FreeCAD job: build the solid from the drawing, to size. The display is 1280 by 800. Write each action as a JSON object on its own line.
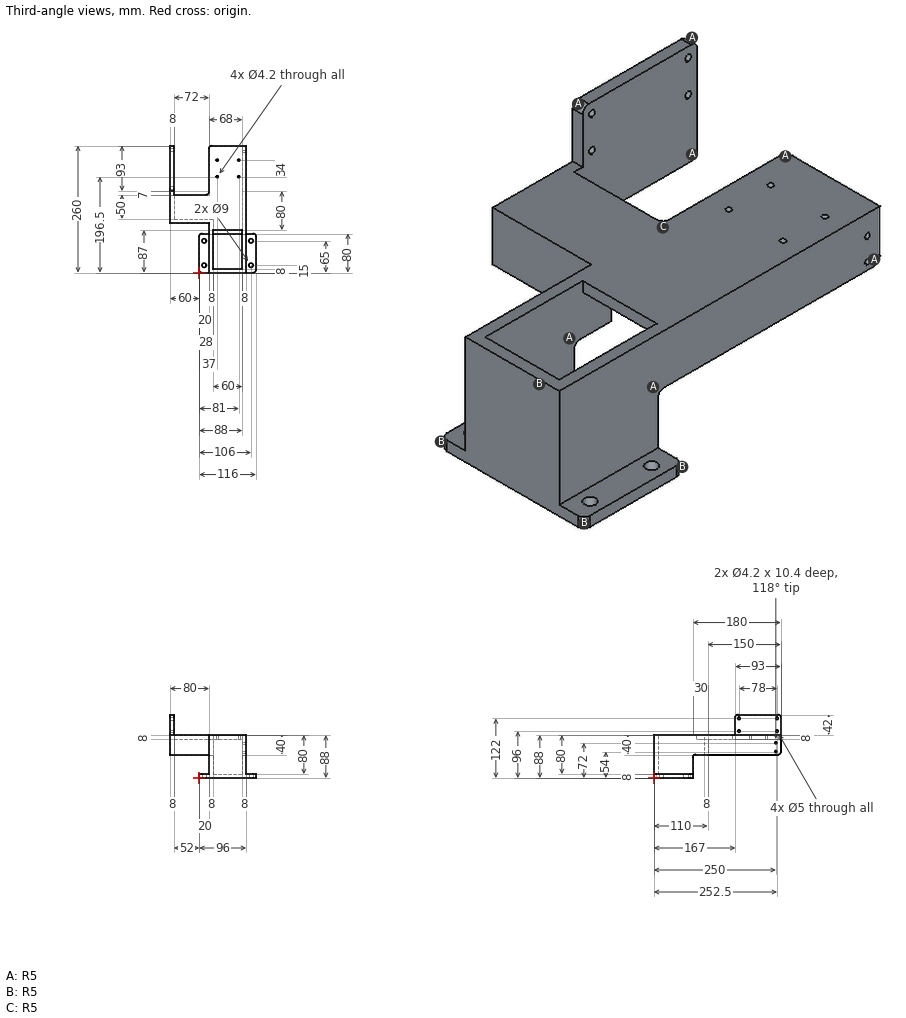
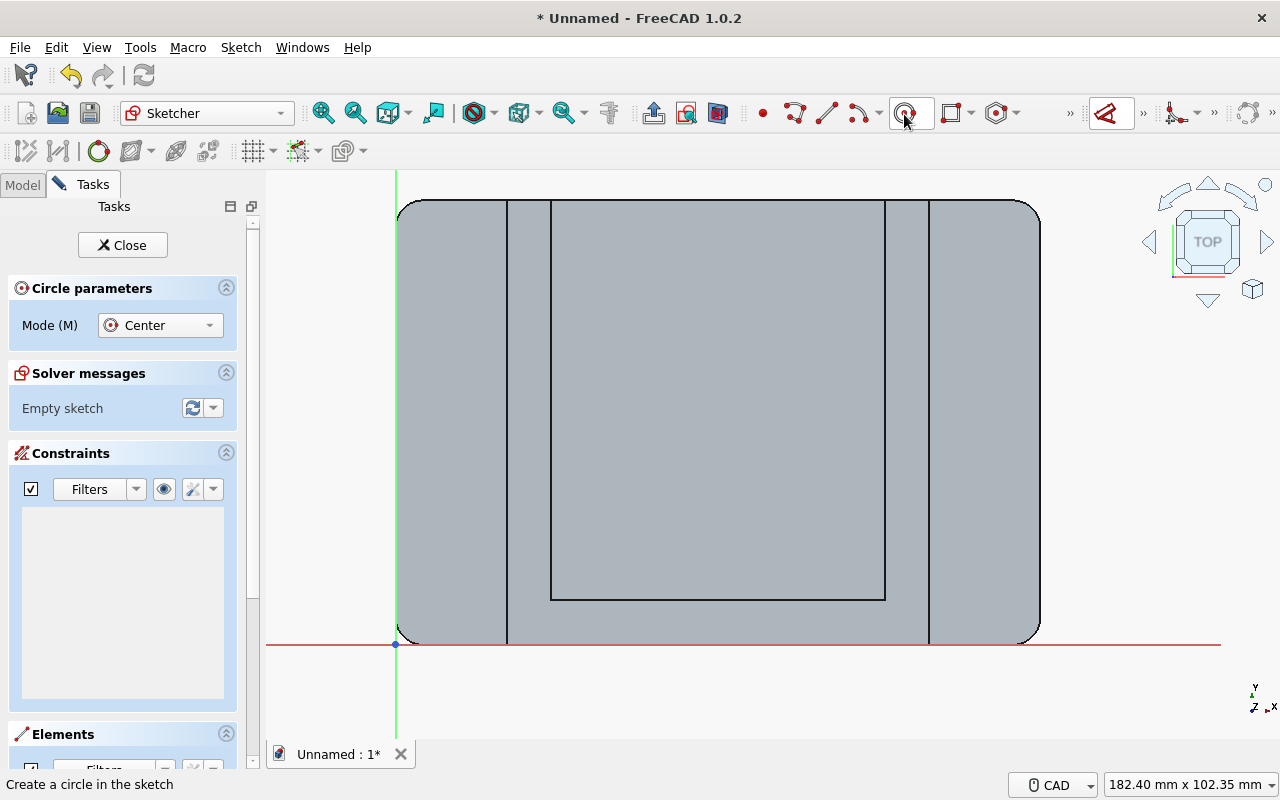
{"action": "left_click", "coordinate": [985, 562]}
{"action": "left_click", "coordinate": [1003, 544]}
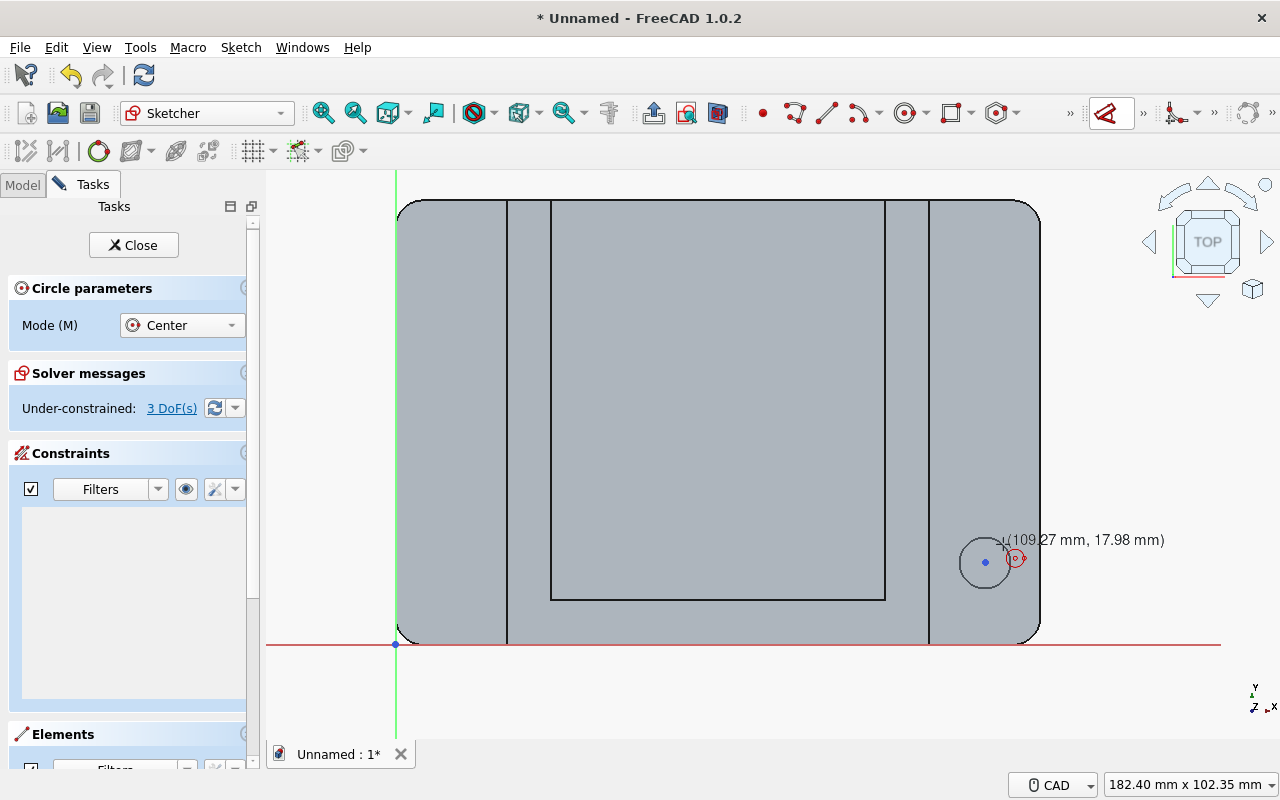
{"action": "left_click", "coordinate": [985, 284]}
{"action": "left_click", "coordinate": [1003, 266]}
{"action": "key", "text": "Escape"}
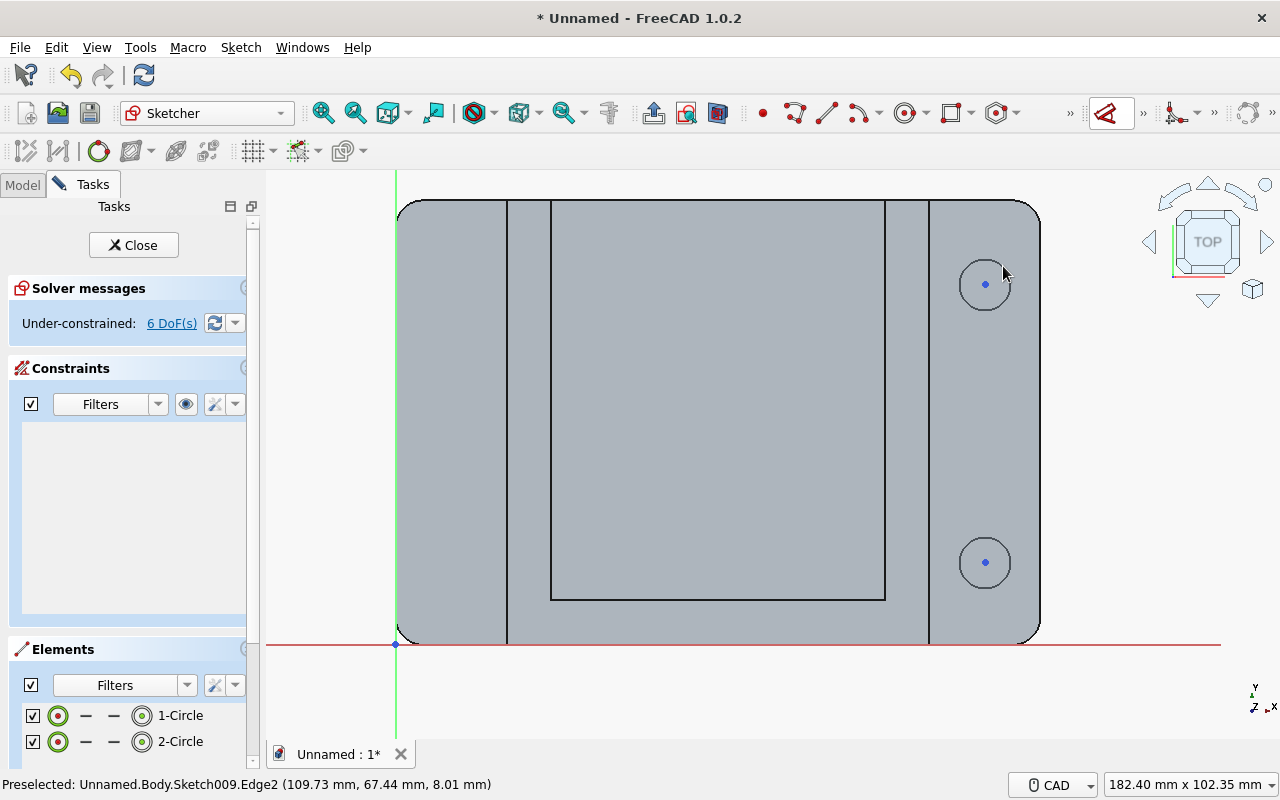
{"action": "left_click", "coordinate": [1003, 545]}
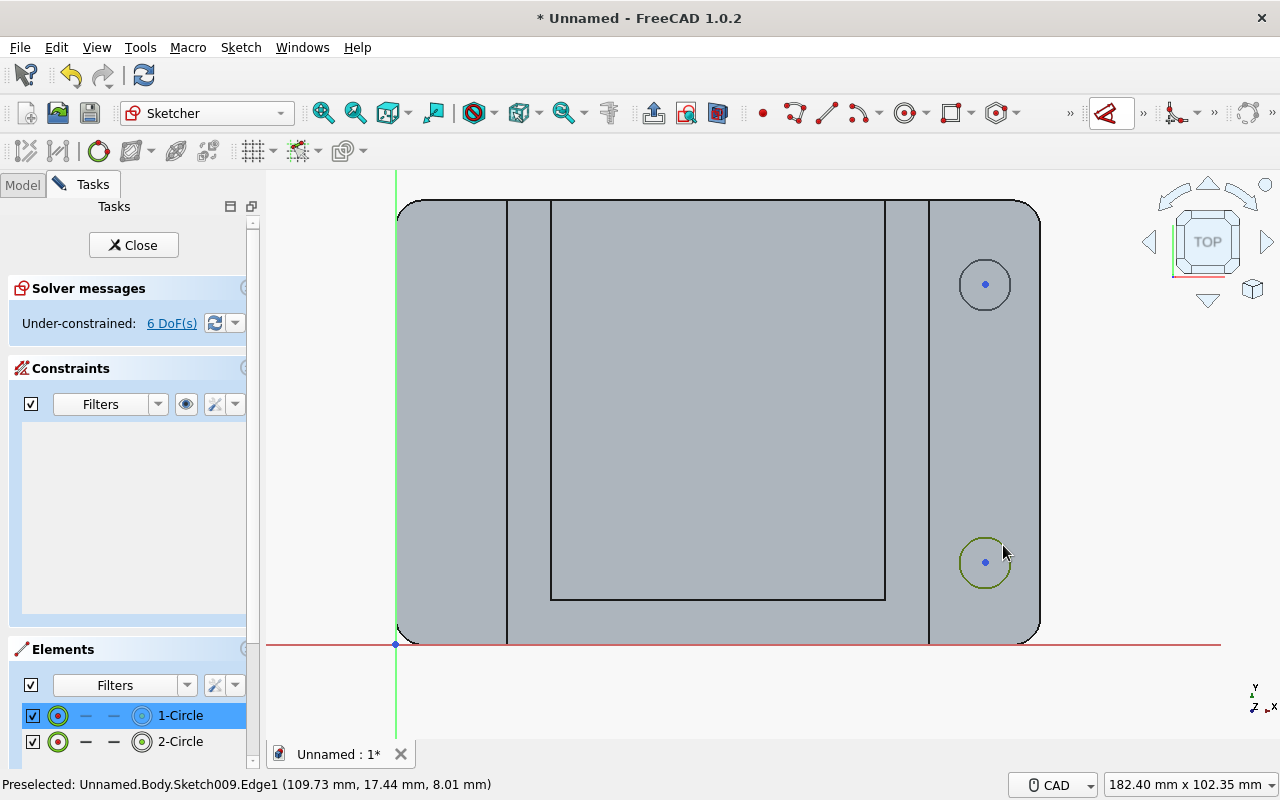
{"action": "left_click", "coordinate": [1003, 267]}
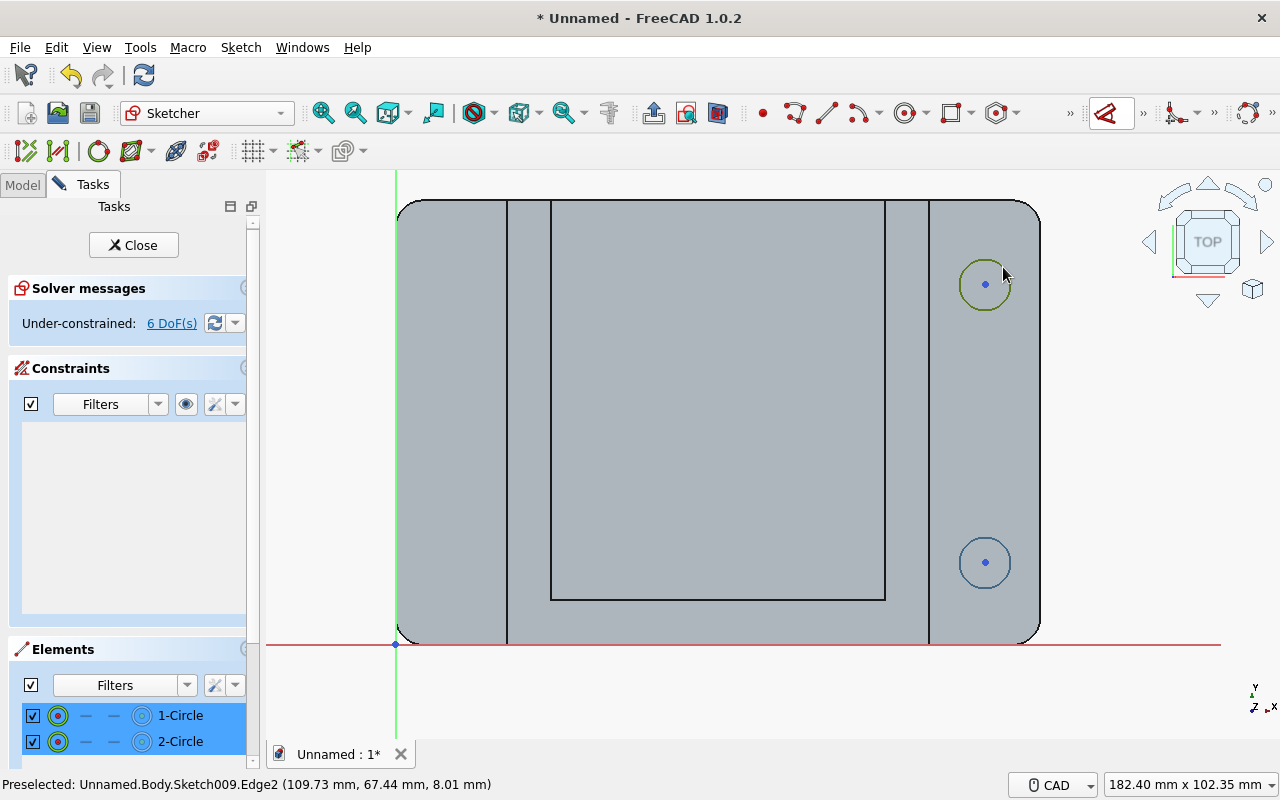
{"action": "key", "text": "e"}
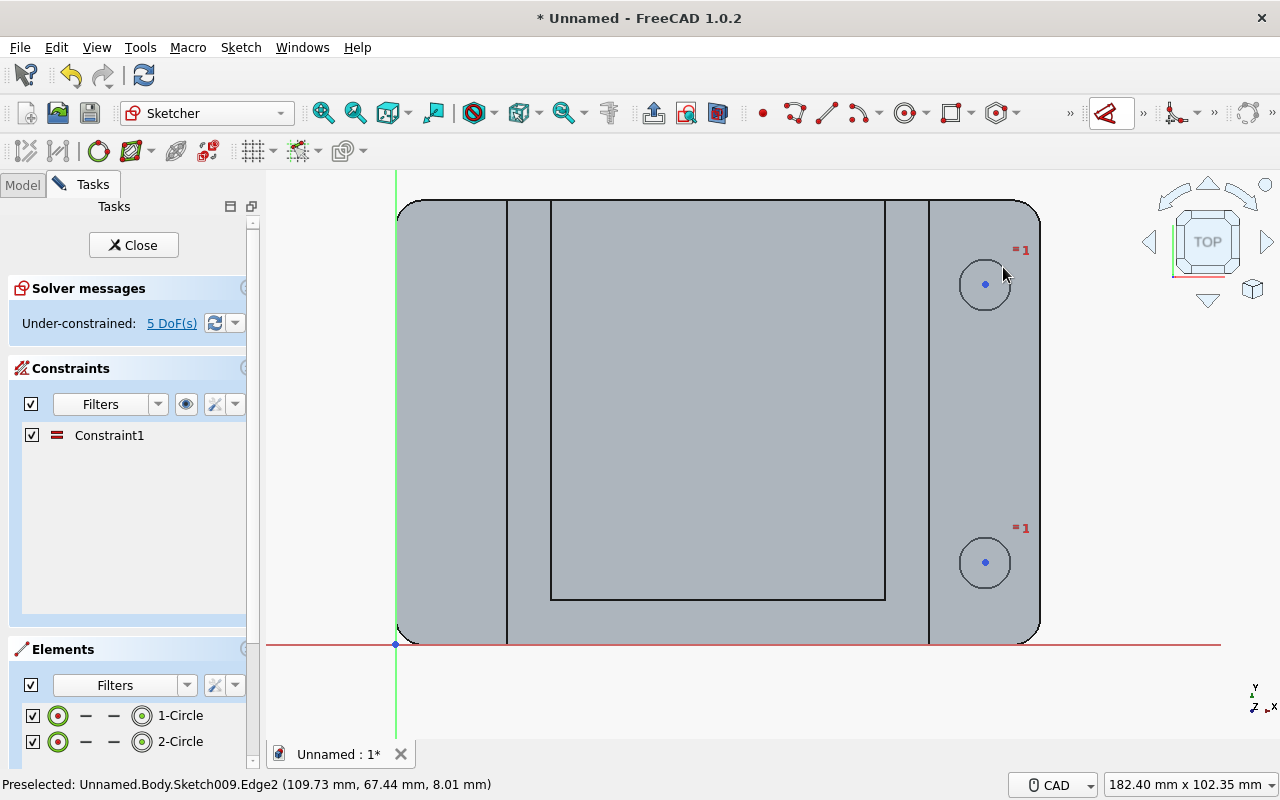
{"action": "left_click", "coordinate": [985, 563]}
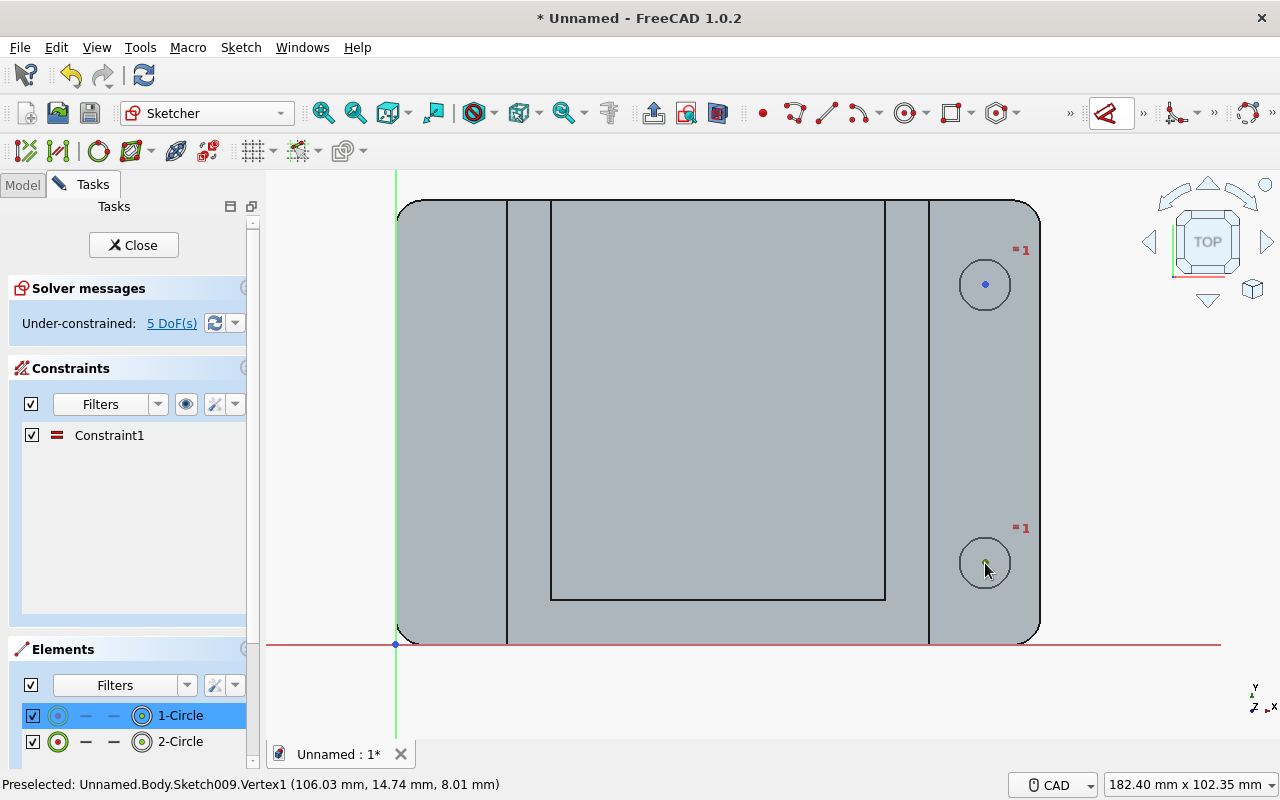
{"action": "left_click", "coordinate": [985, 285]}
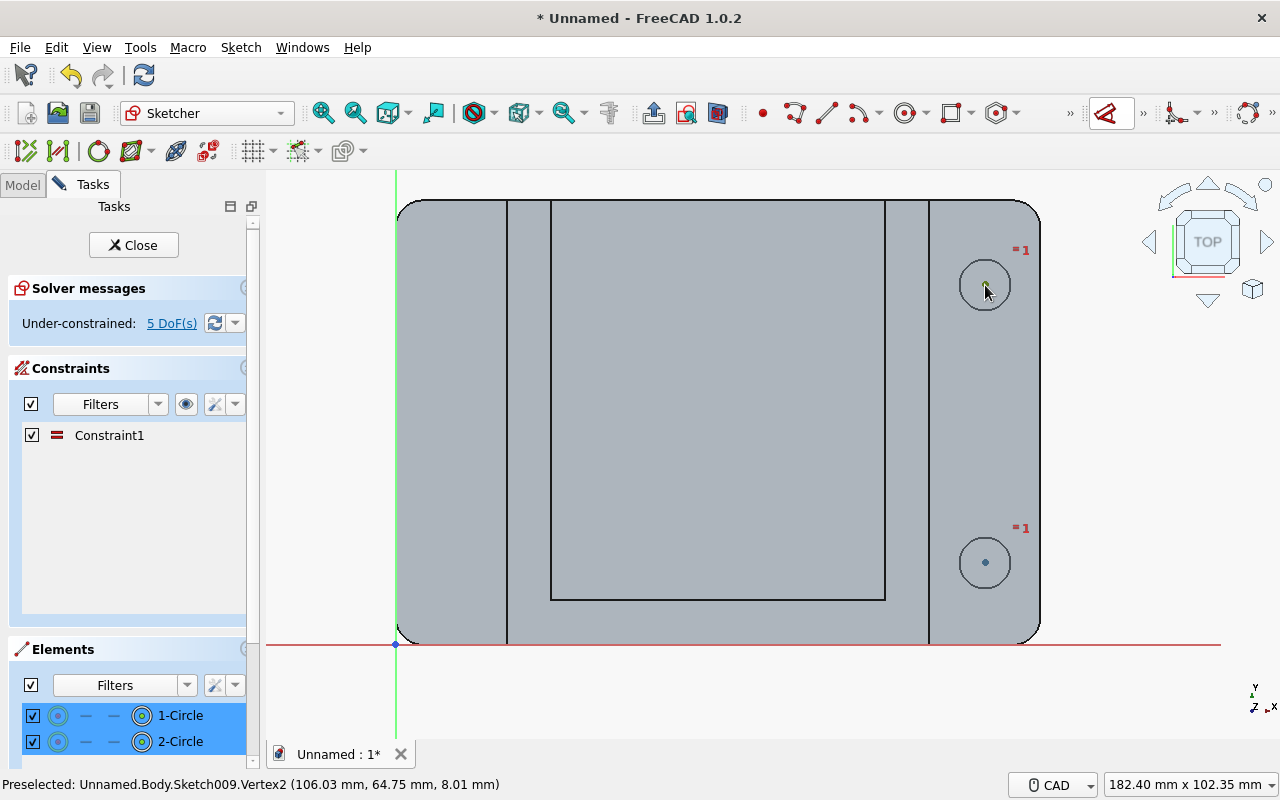
{"action": "key", "text": "v"}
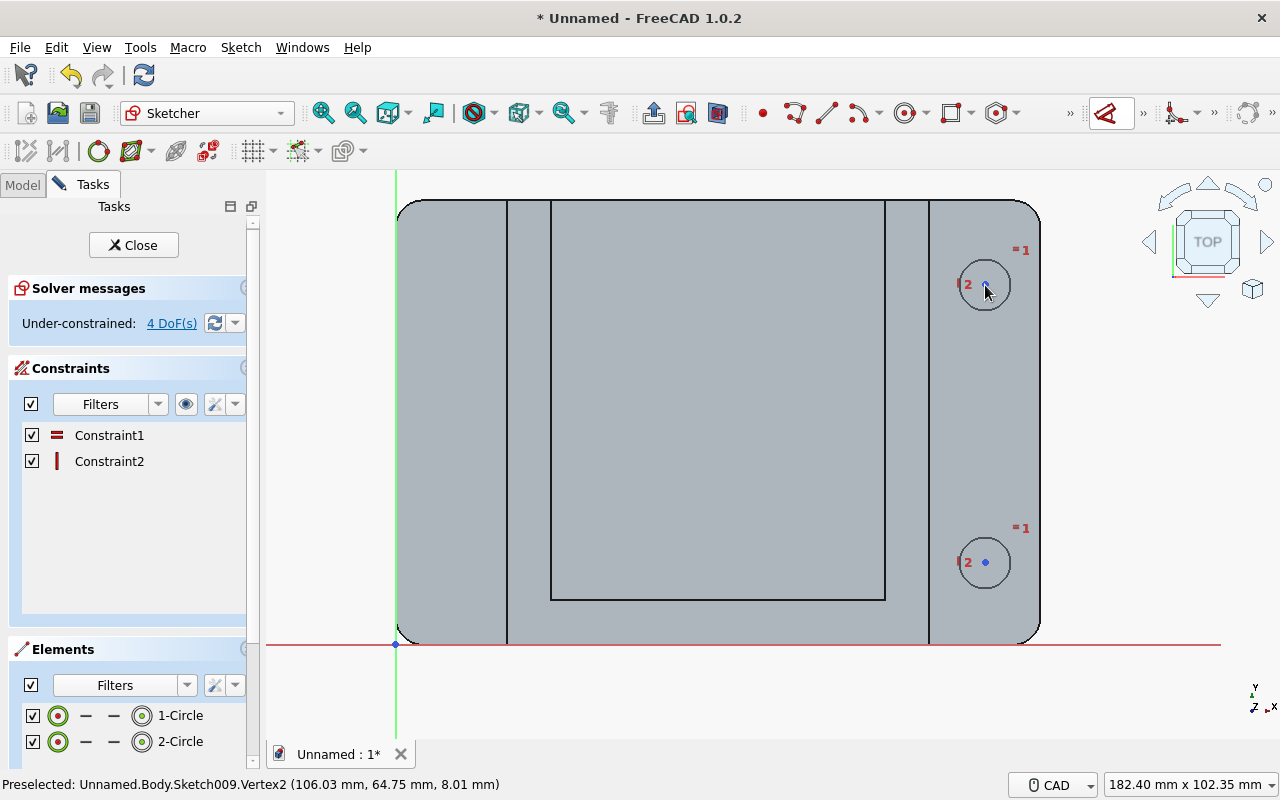
{"action": "left_click", "coordinate": [1003, 545]}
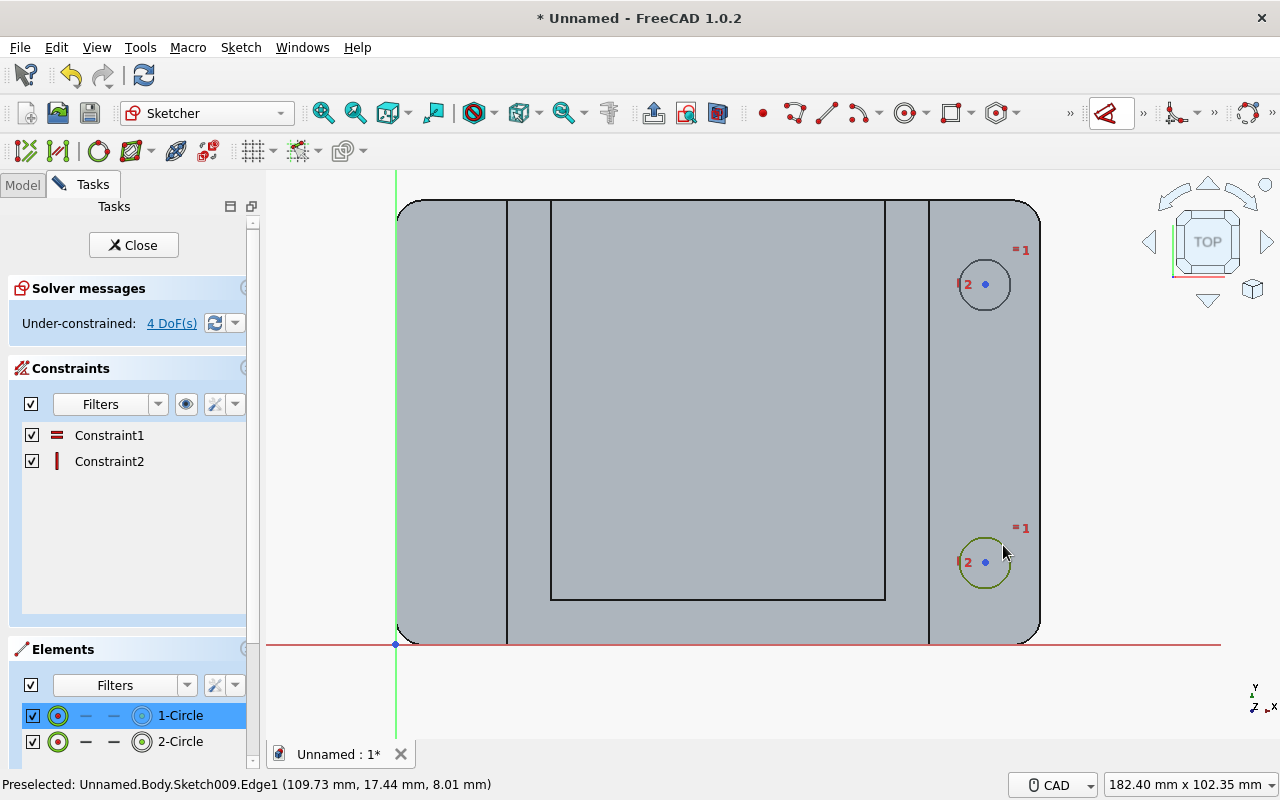
{"action": "left_click", "coordinate": [1128, 114]}